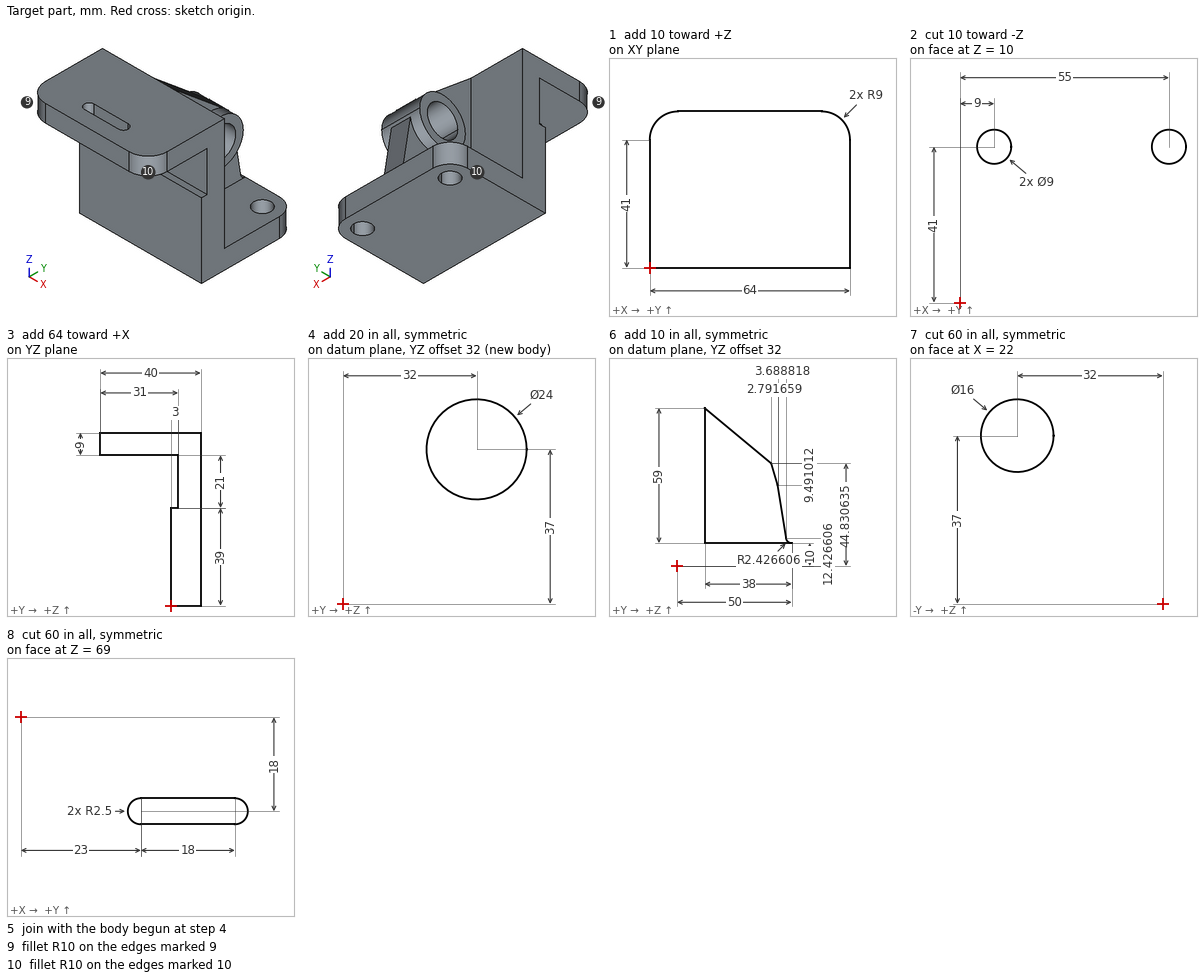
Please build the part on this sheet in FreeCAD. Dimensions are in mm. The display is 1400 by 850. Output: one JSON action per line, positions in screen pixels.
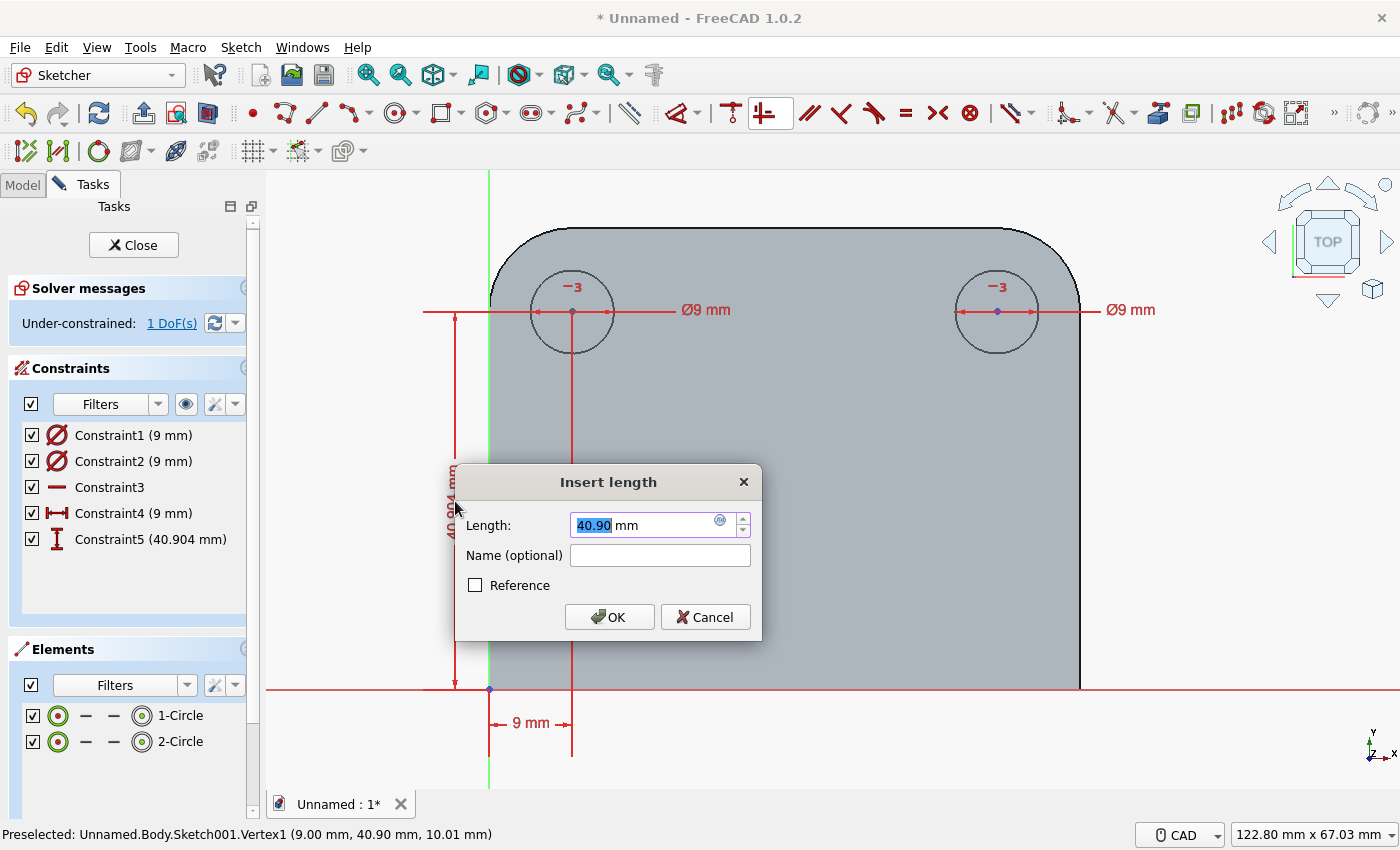
{"action": "type", "text": "41"}
{"action": "key", "text": "Return"}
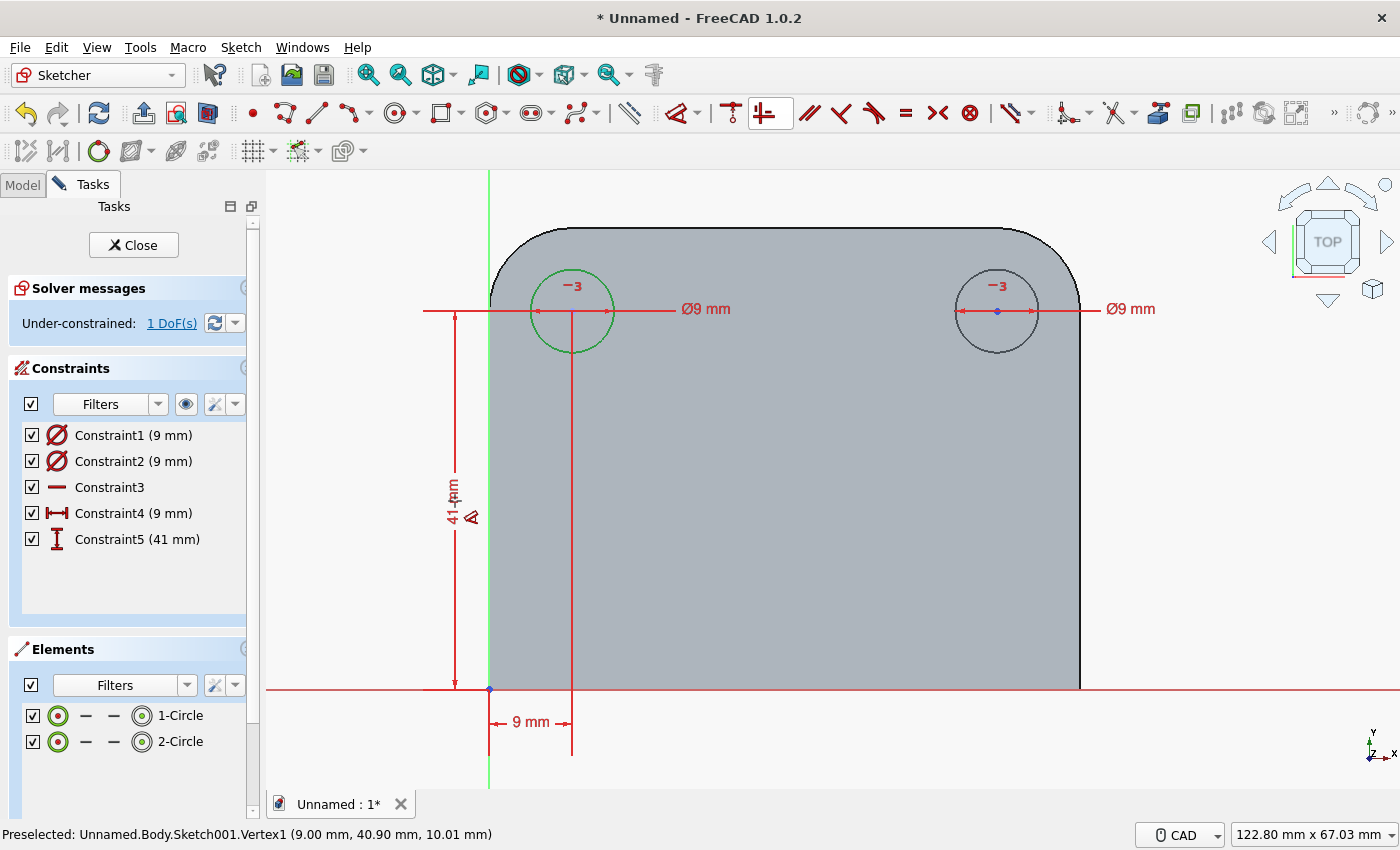
{"action": "left_click", "coordinate": [997, 311]}
{"action": "left_click", "coordinate": [743, 724]}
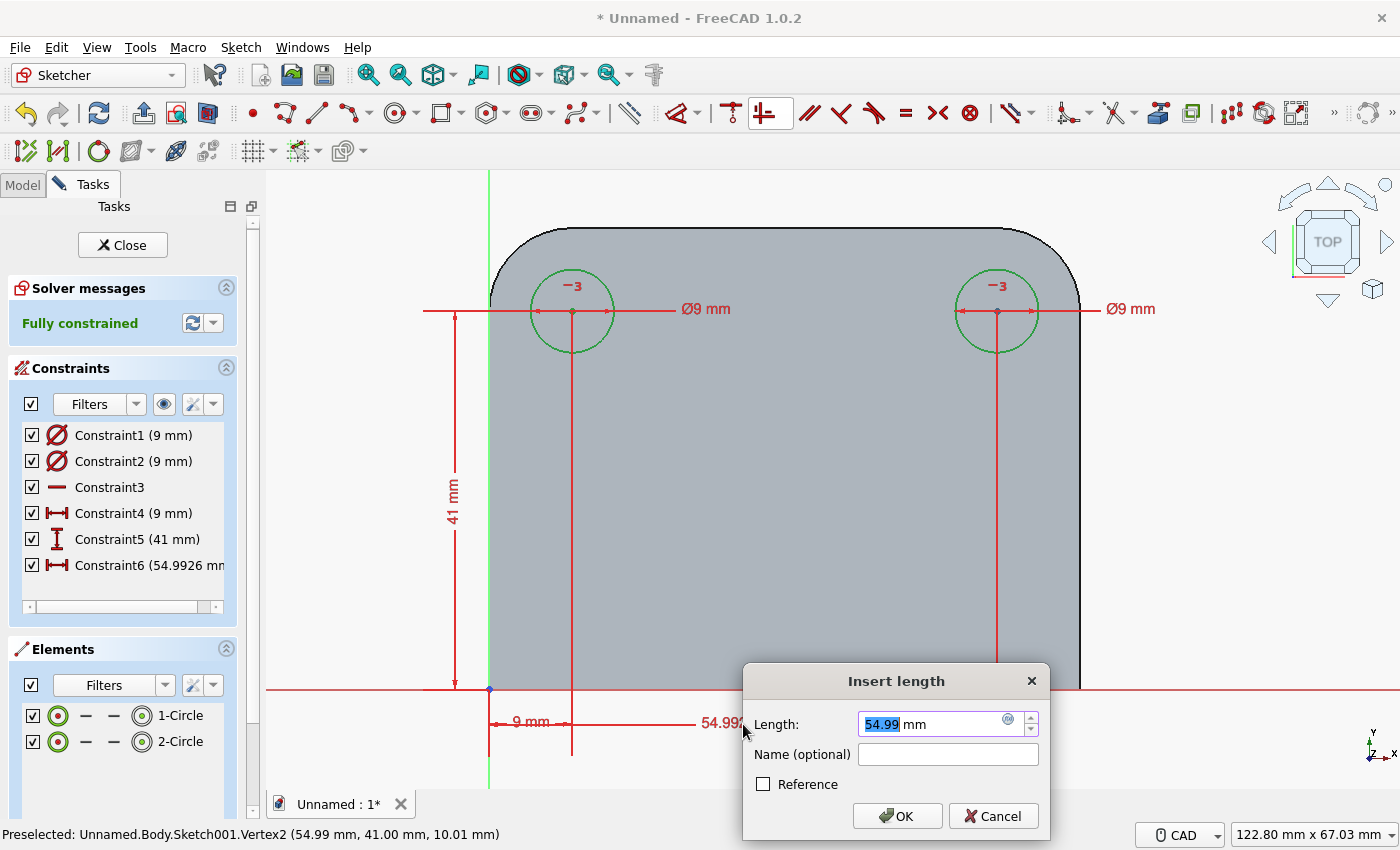
{"action": "type", "text": "55"}
{"action": "key", "text": "Return"}
{"action": "key", "text": "Escape"}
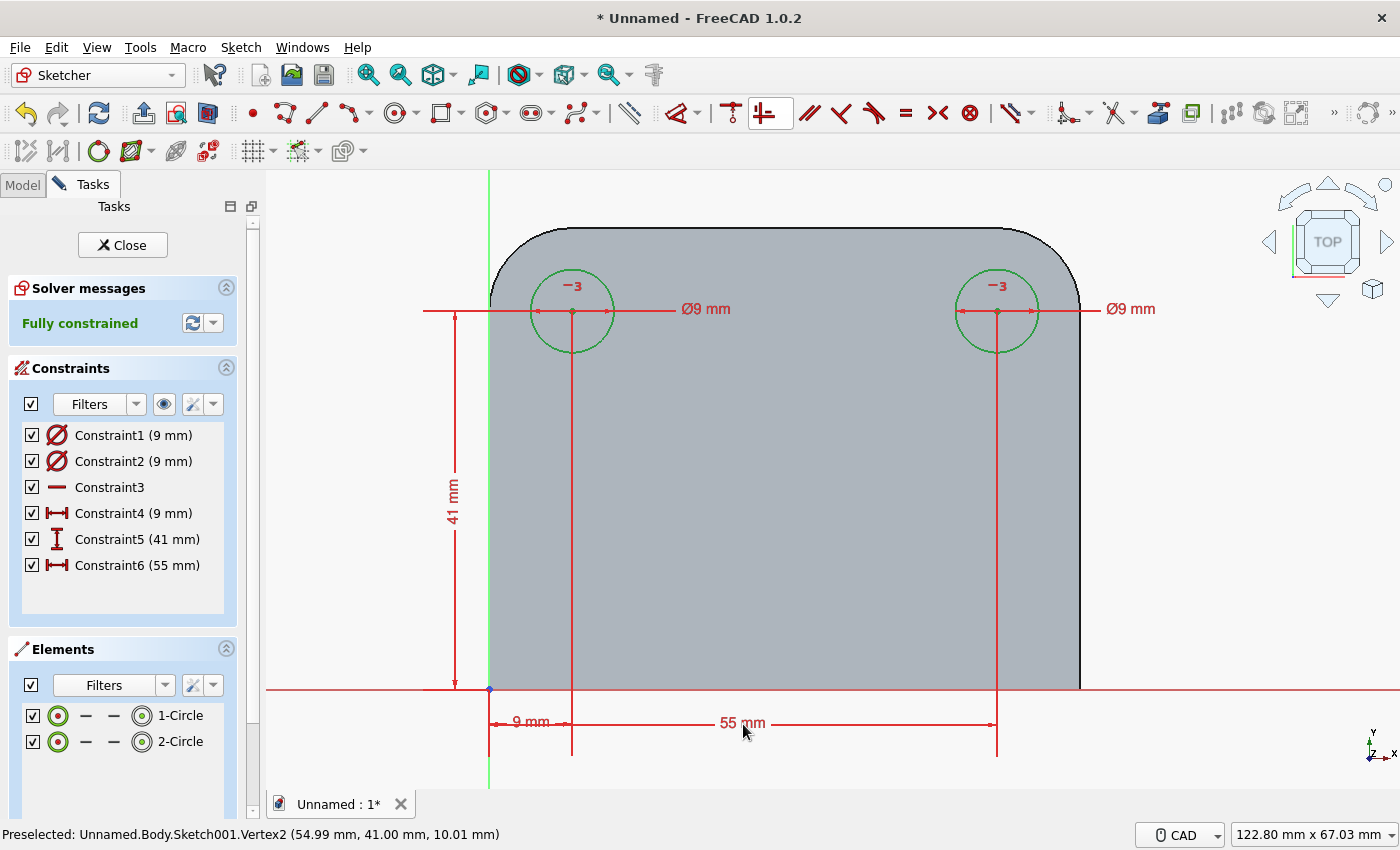
{"action": "left_click", "coordinate": [123, 245]}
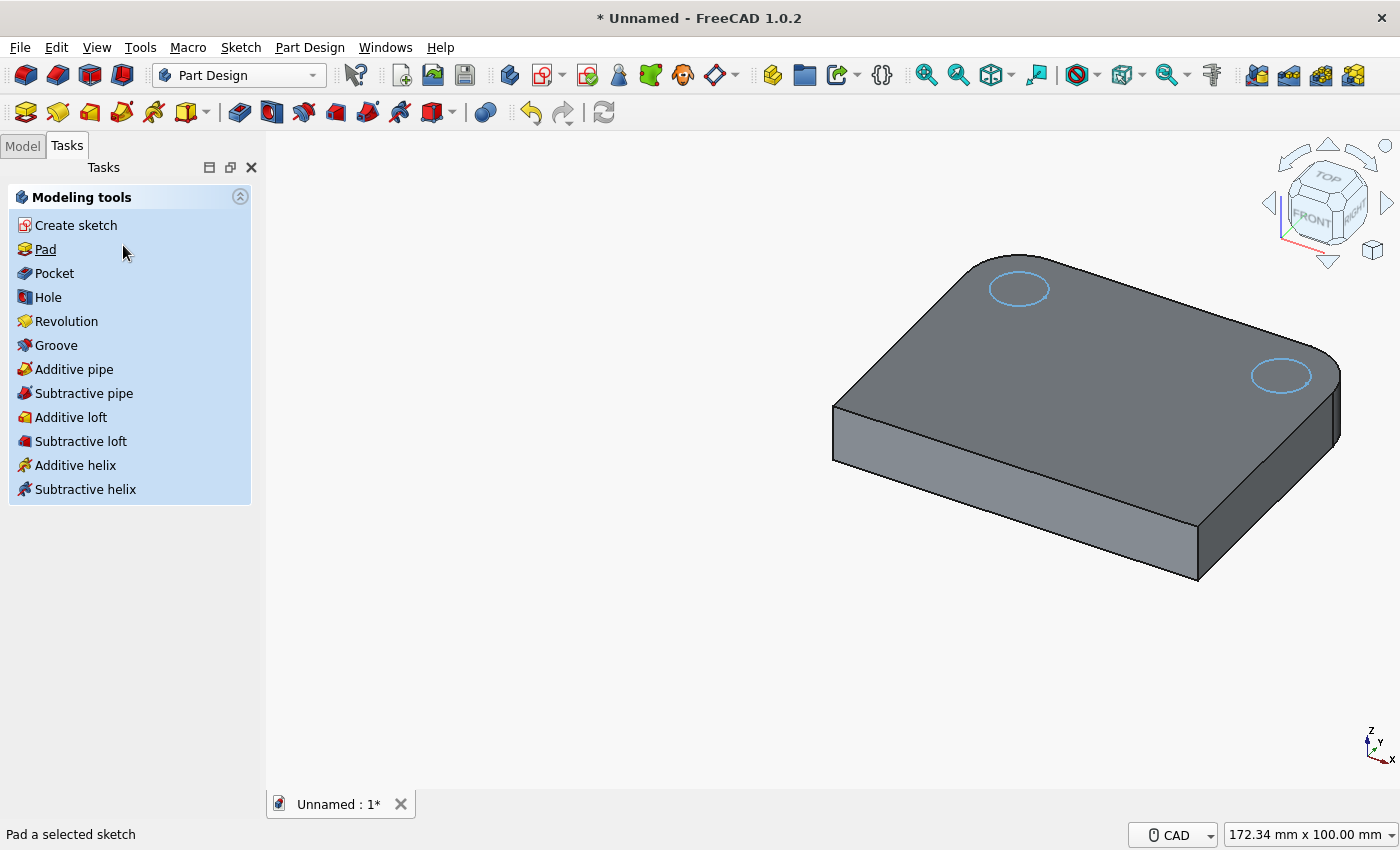
{"action": "left_click", "coordinate": [240, 112]}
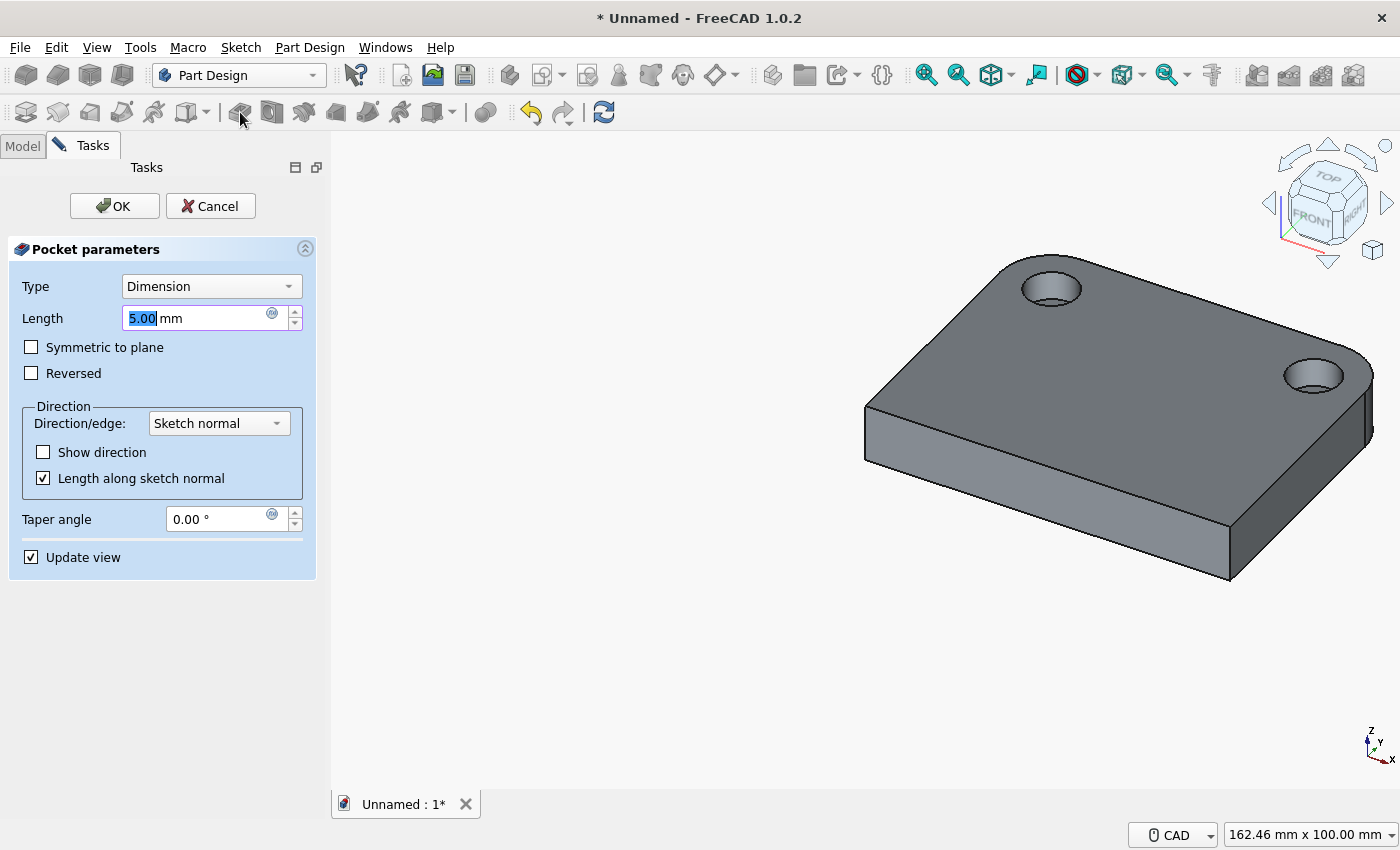
{"action": "type", "text": "10"}
{"action": "key", "text": "Tab"}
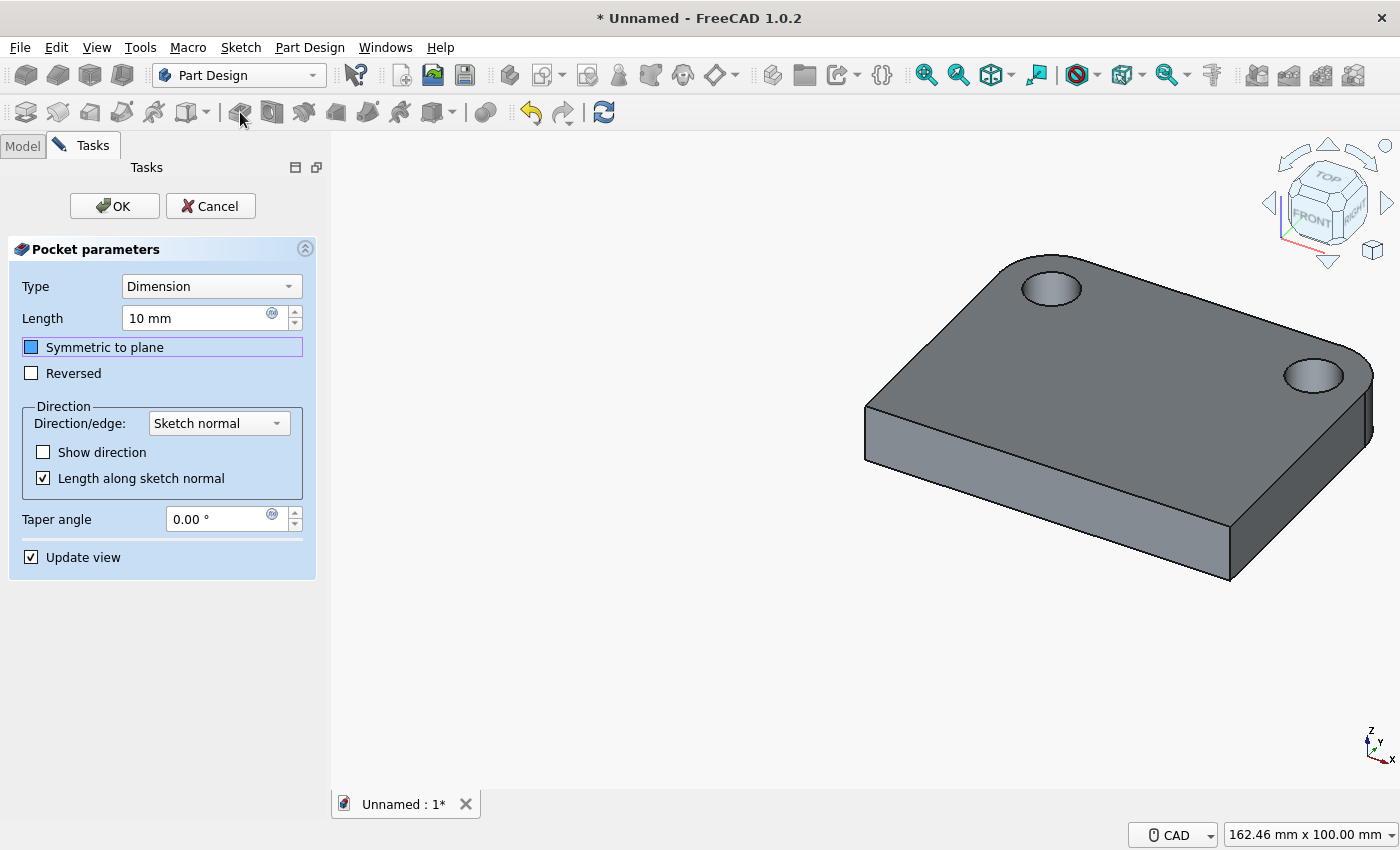
{"action": "left_click", "coordinate": [115, 206]}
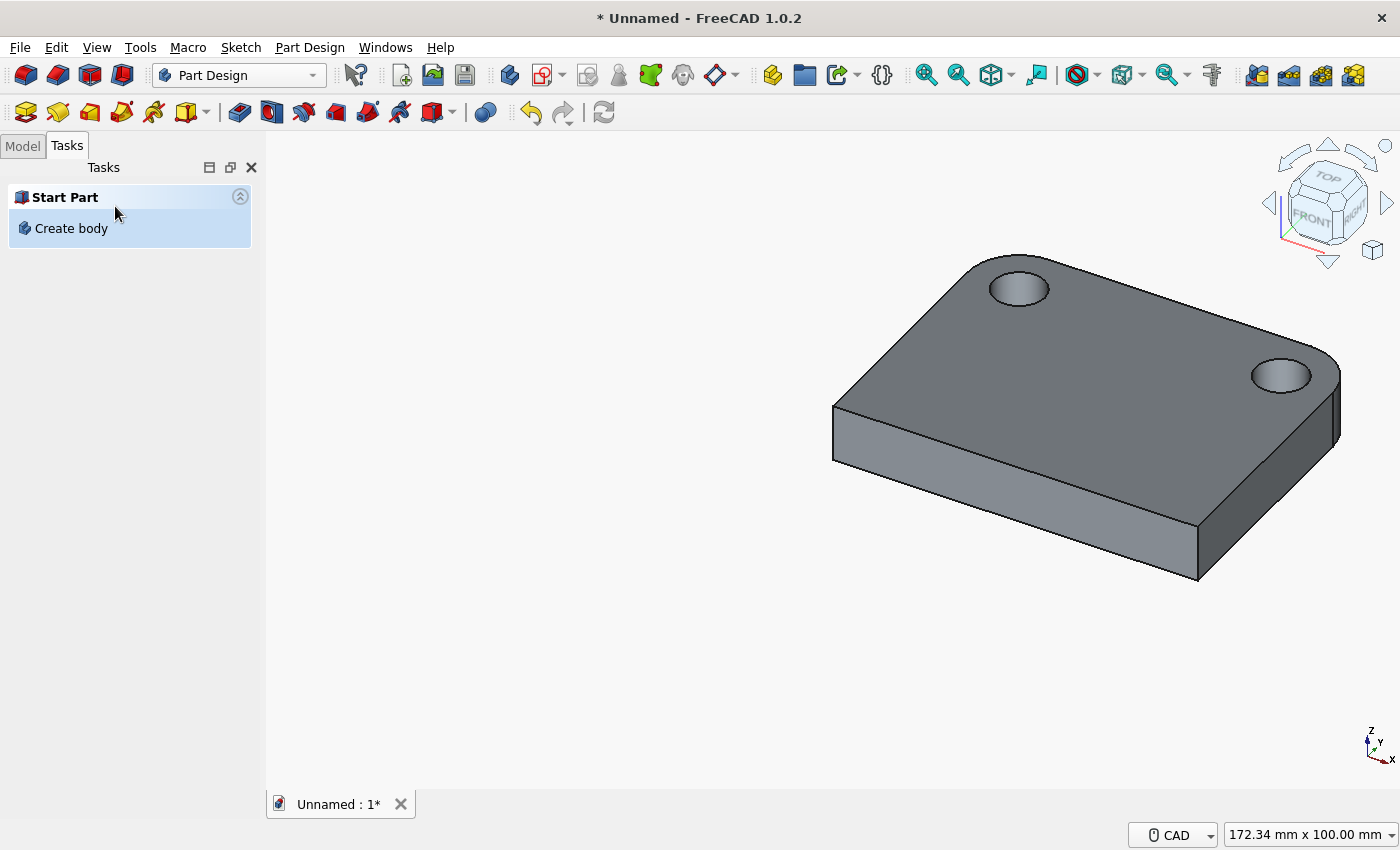
{"action": "left_click", "coordinate": [542, 76]}